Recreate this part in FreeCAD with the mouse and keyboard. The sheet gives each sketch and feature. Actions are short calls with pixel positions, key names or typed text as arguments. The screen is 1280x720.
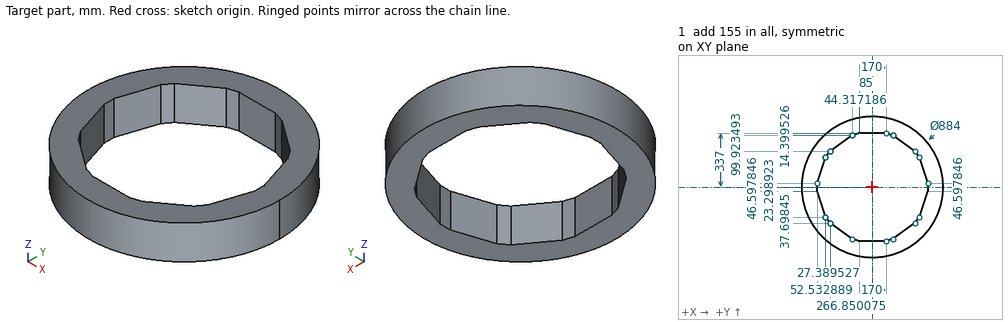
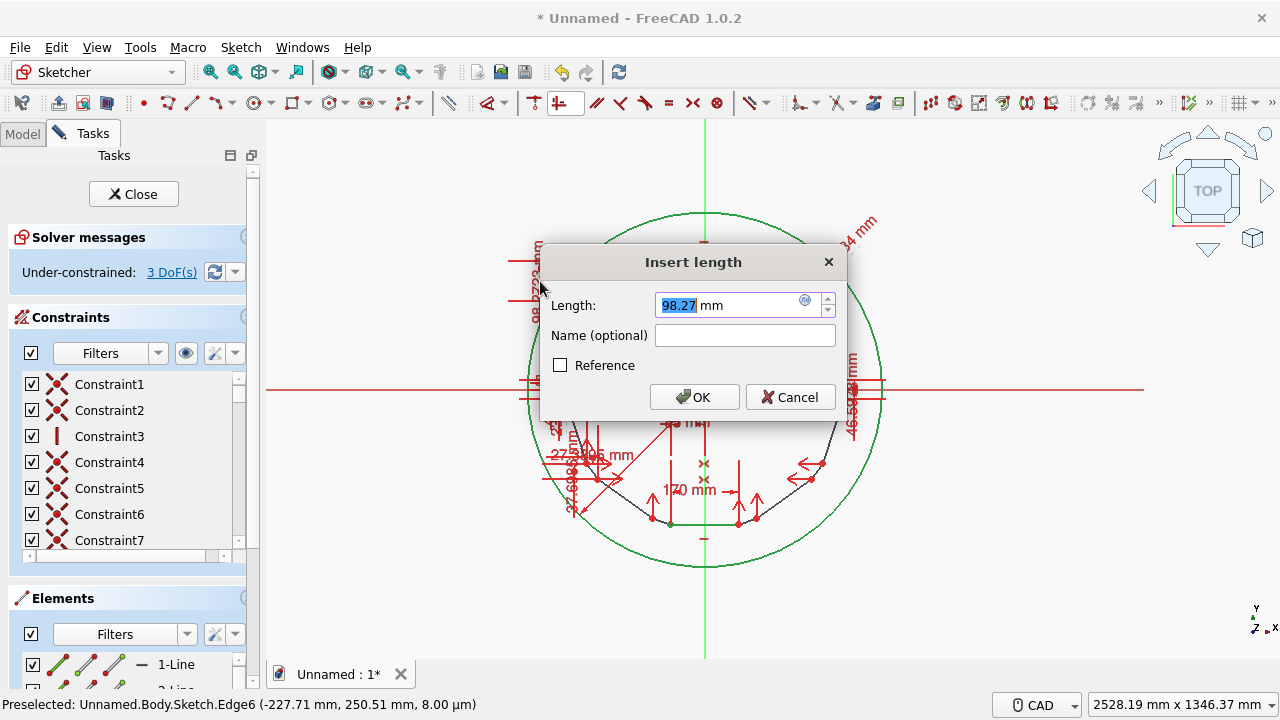
text(99.923493)
key(Return)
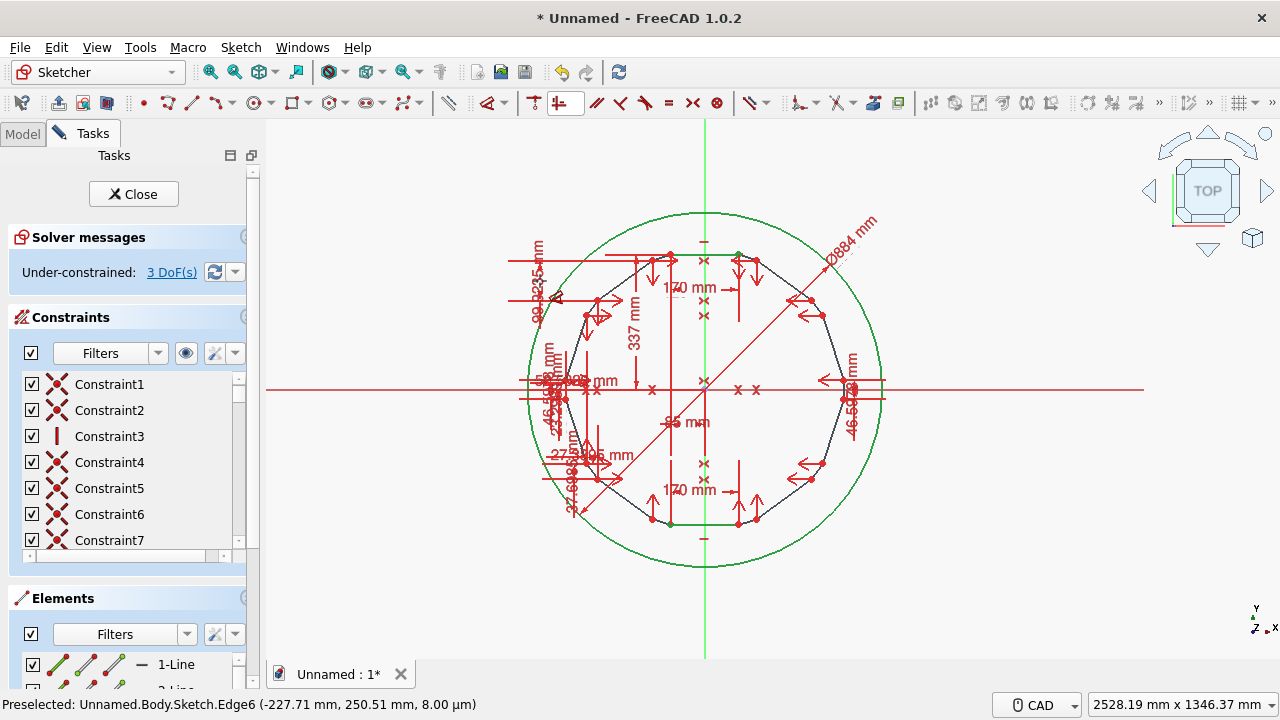
scroll(662, 258, up, 5)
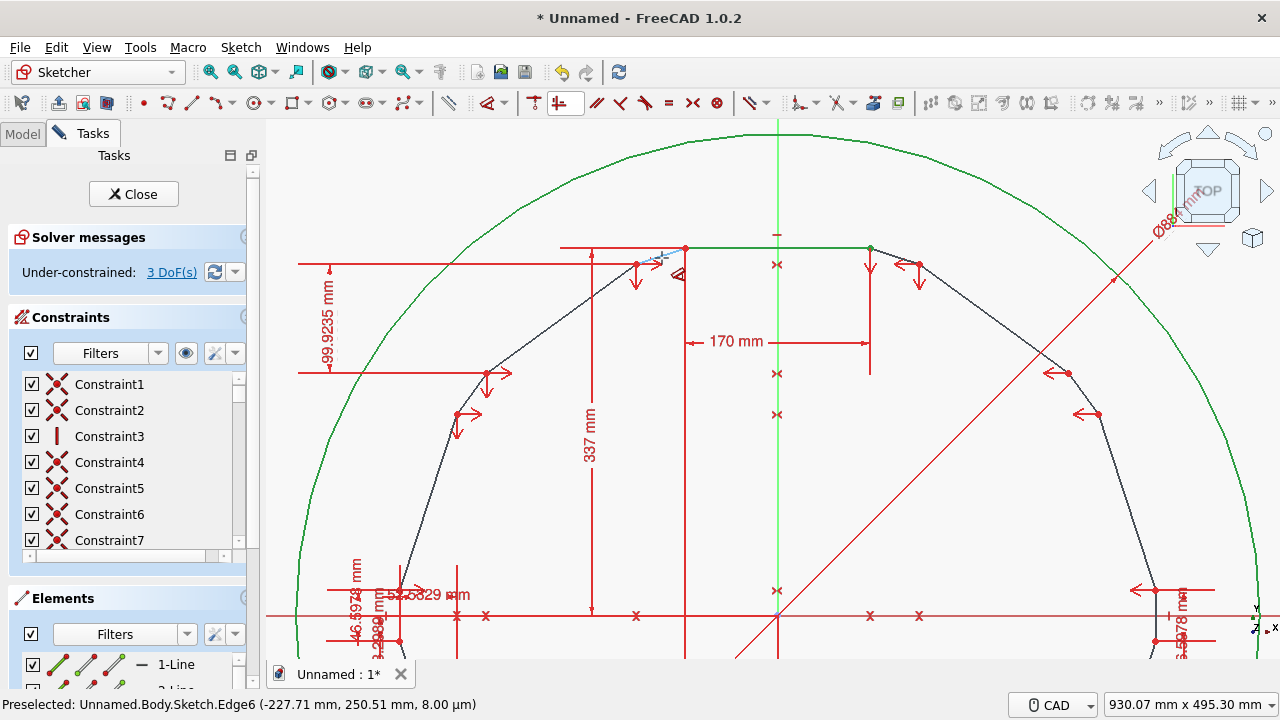
click(661, 256)
click(661, 214)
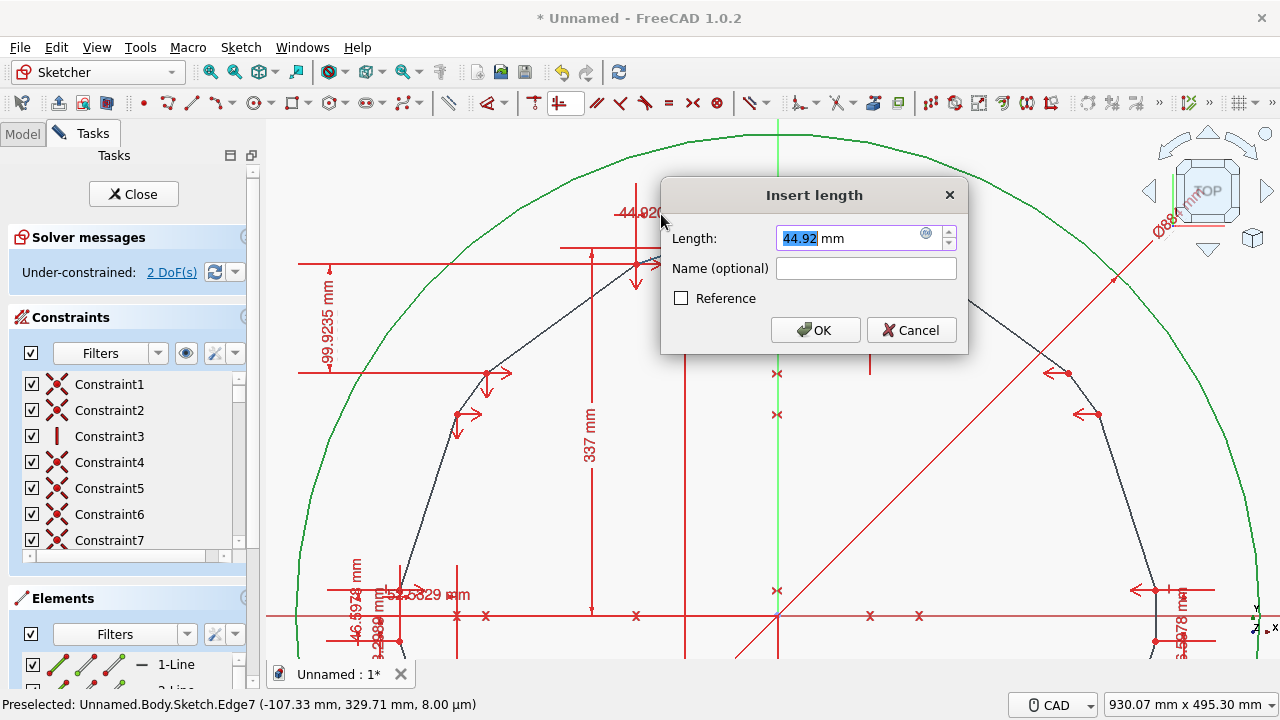
text(44.317186)
key(Return)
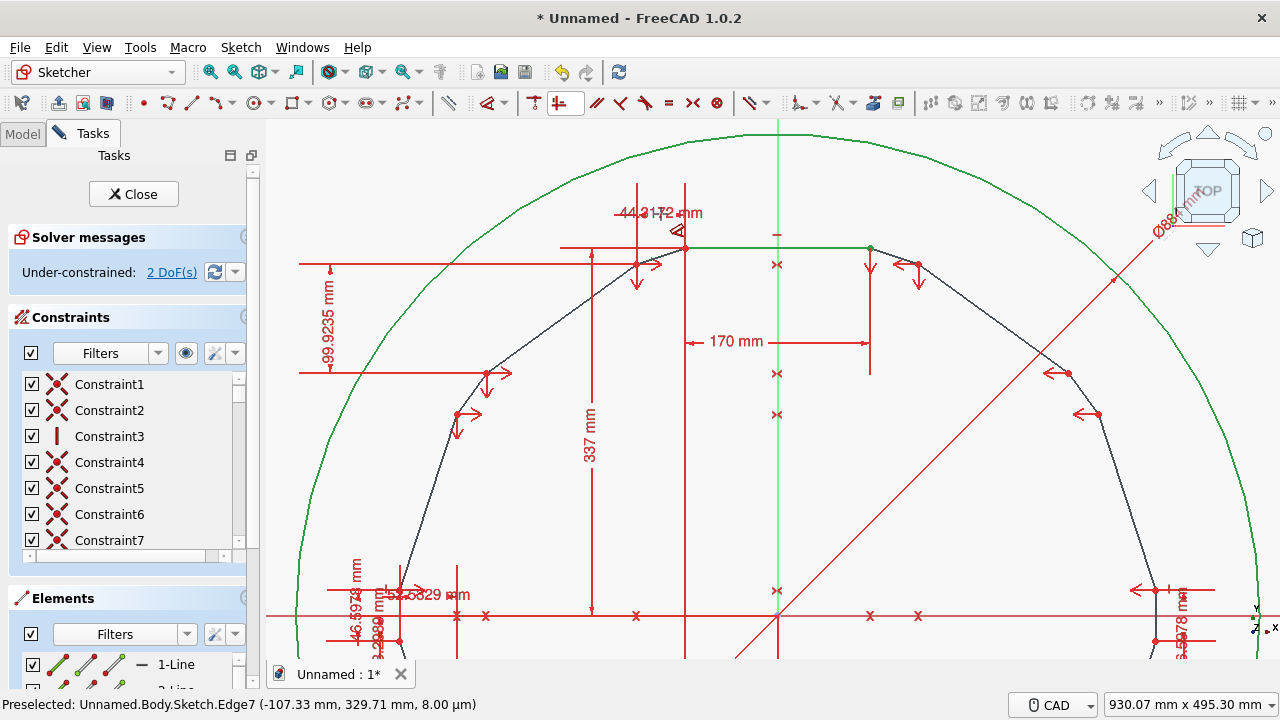
scroll(651, 260, up, 5)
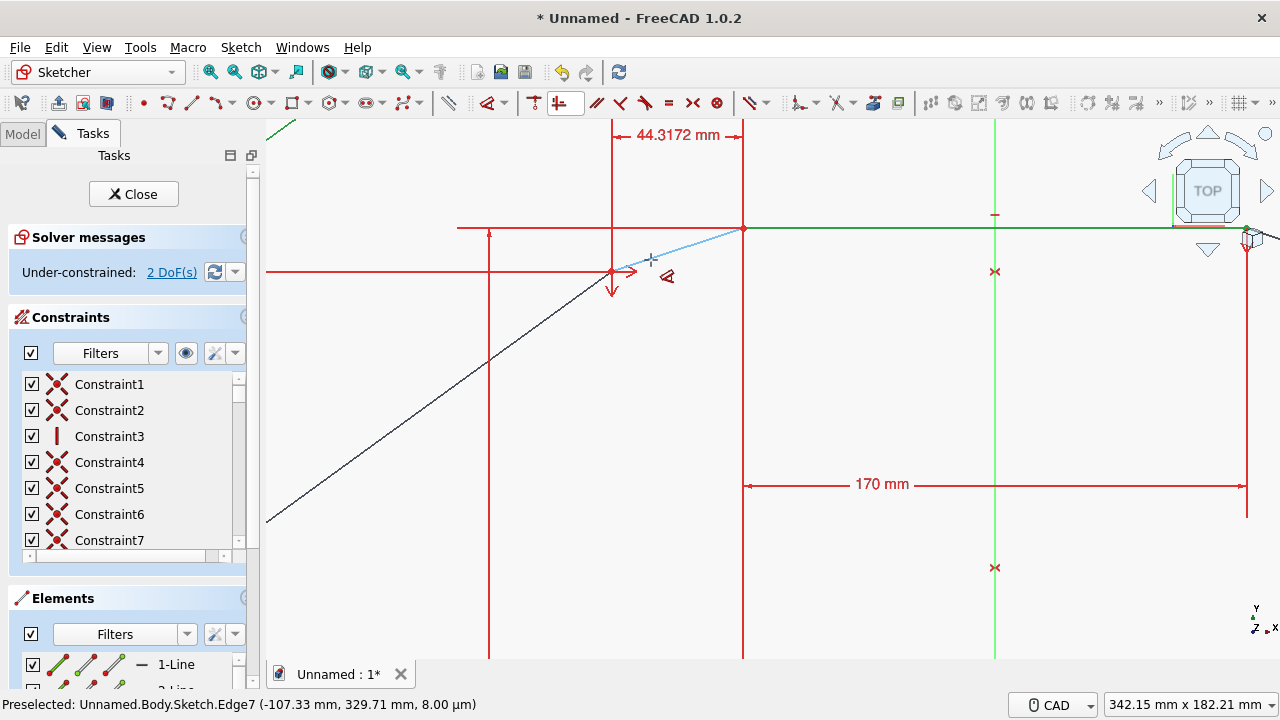
click(651, 259)
click(578, 250)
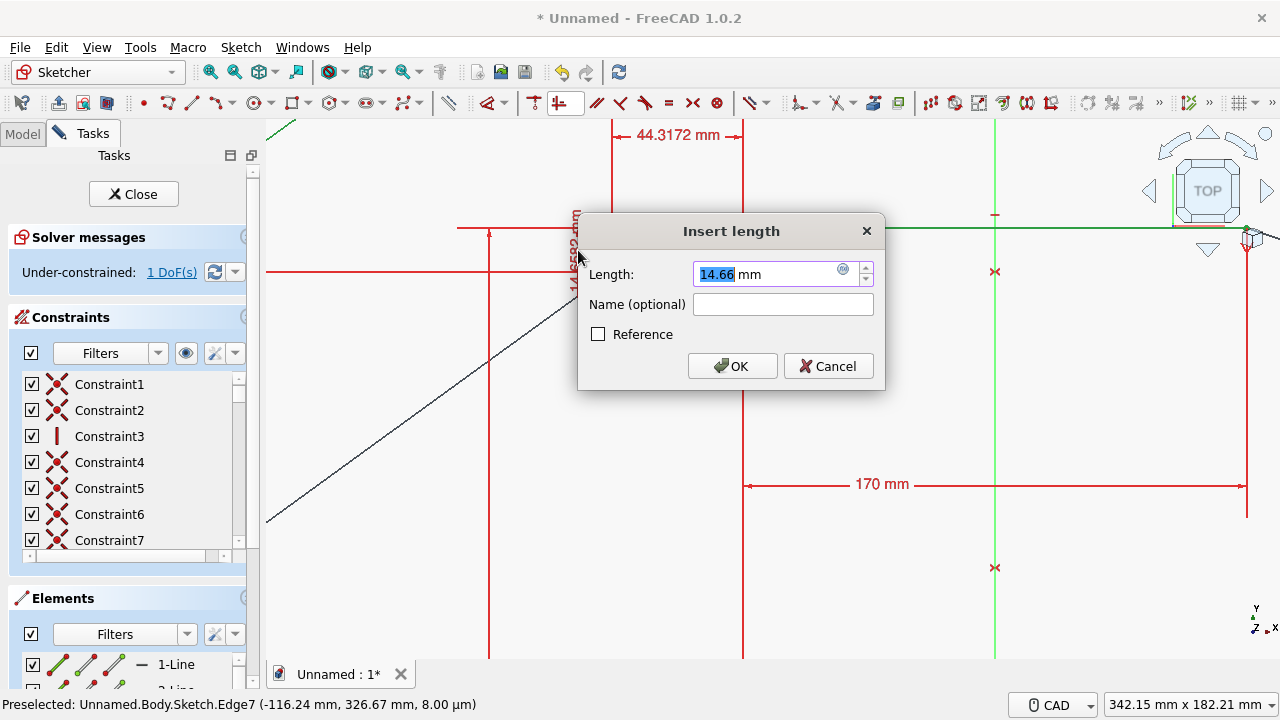
text(14.399526)
key(Return)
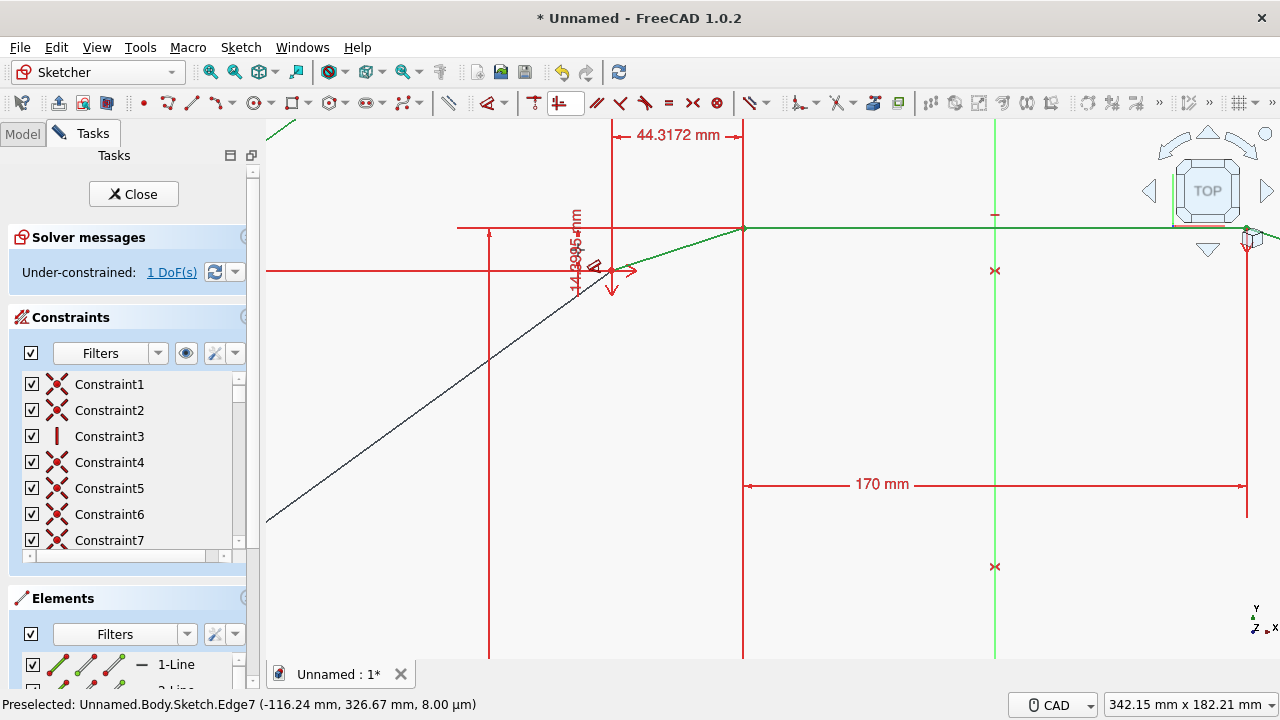
scroll(659, 258, down, 10)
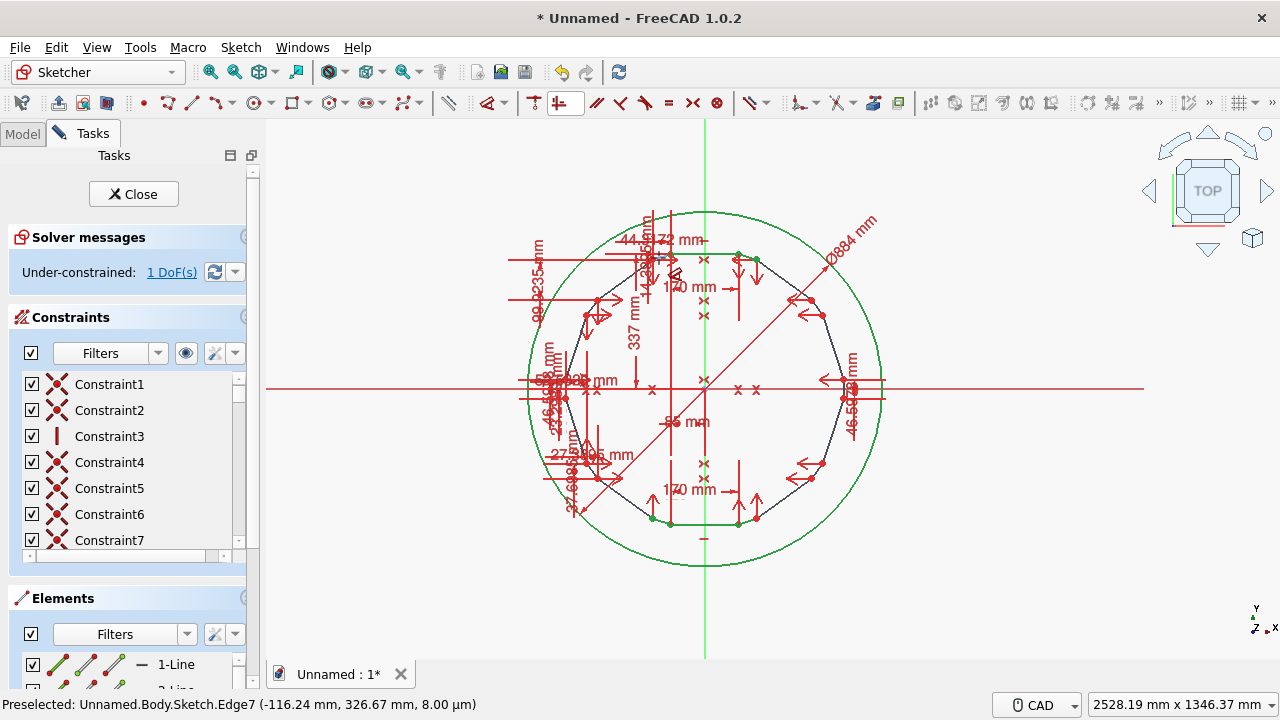
click(598, 479)
click(614, 513)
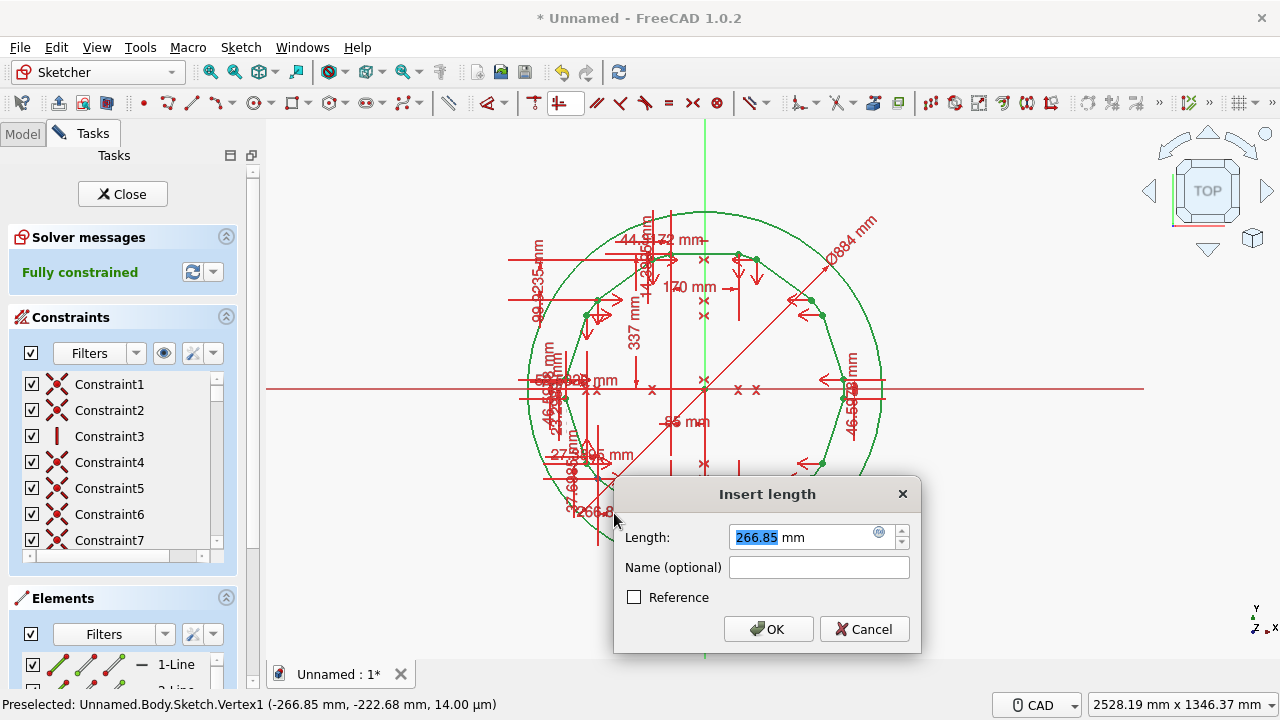
text(266.850075)
key(Return)
key(Escape)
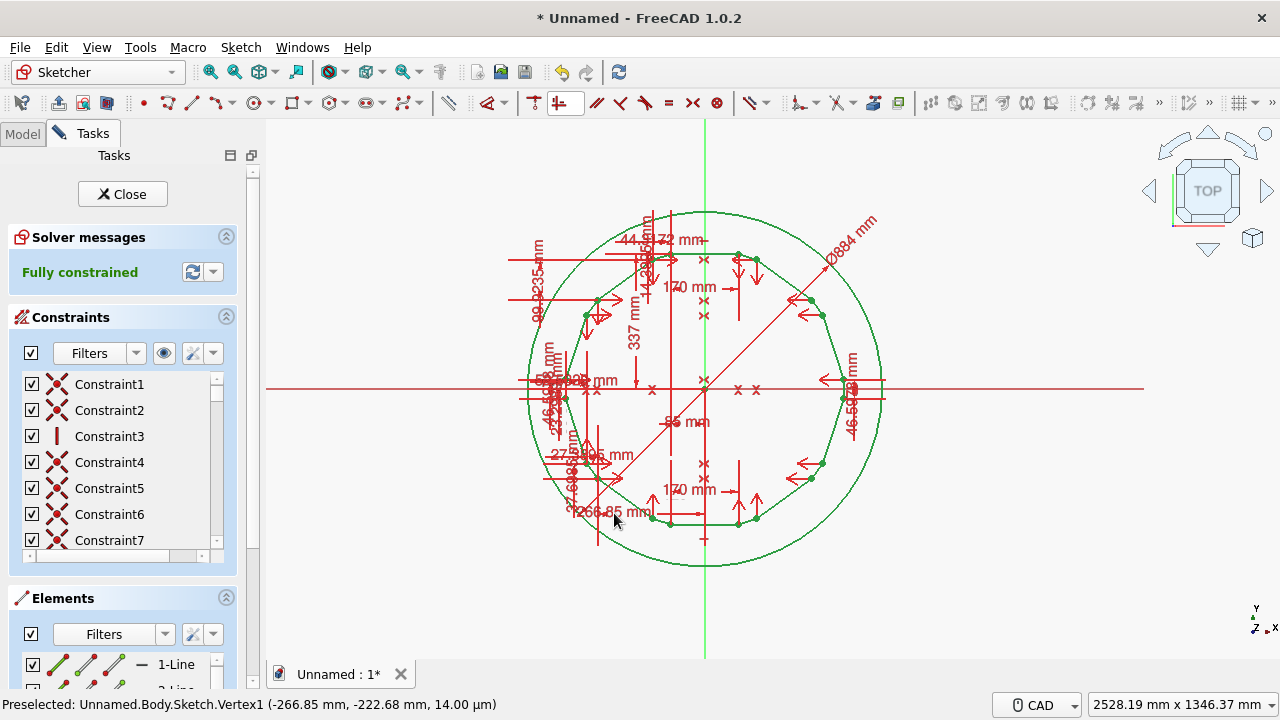
click(123, 194)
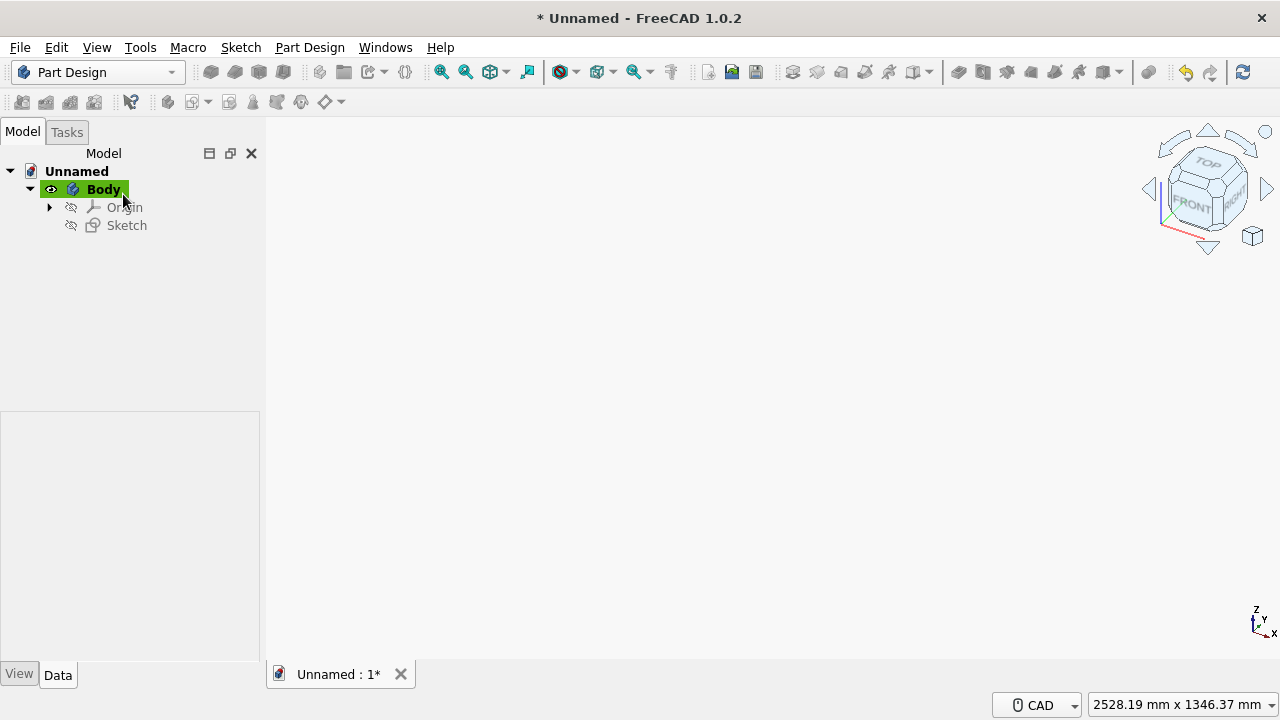
click(794, 72)